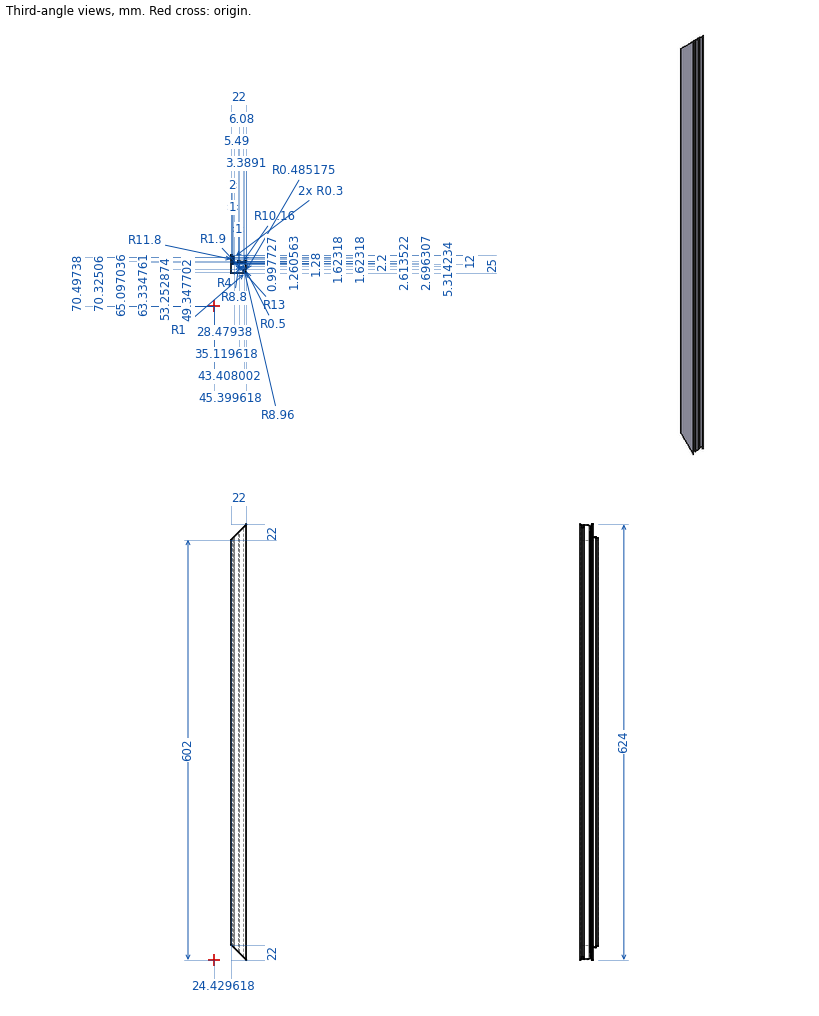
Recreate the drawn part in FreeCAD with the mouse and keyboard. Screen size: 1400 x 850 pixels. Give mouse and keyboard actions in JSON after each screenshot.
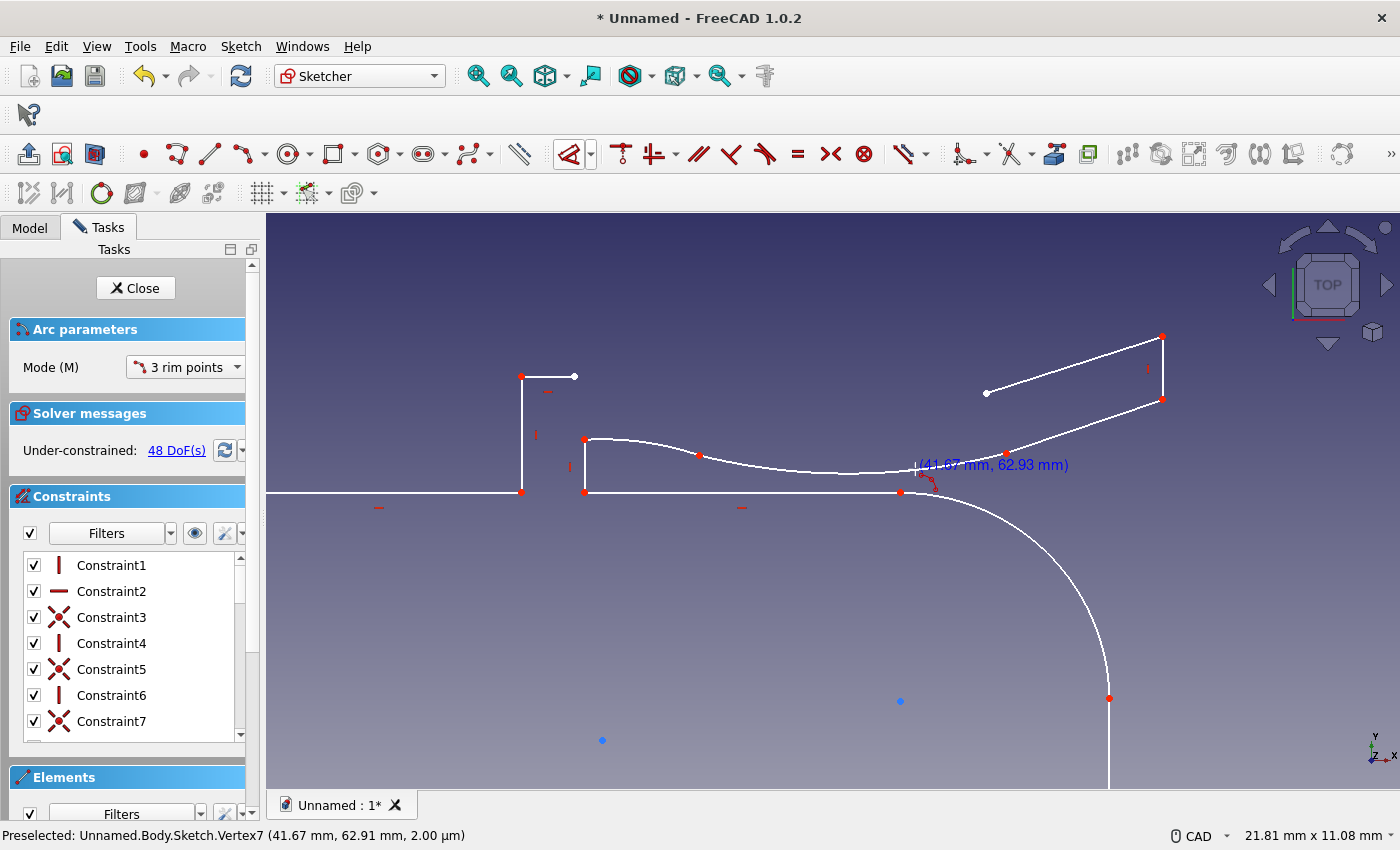
{"action": "left_click", "coordinate": [987, 393]}
{"action": "left_click", "coordinate": [717, 394]}
{"action": "left_click", "coordinate": [852, 412]}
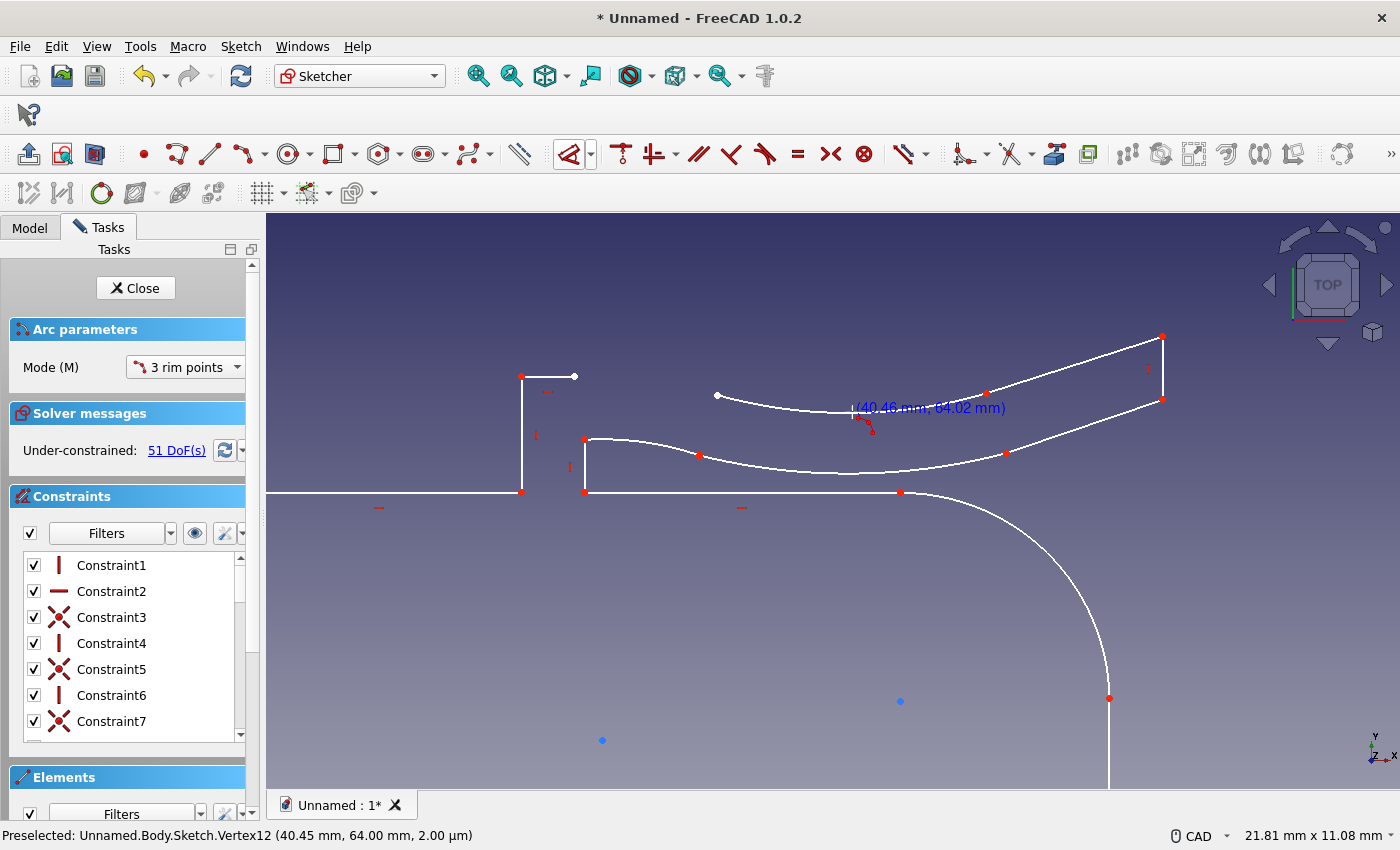
{"action": "left_click", "coordinate": [717, 395]}
{"action": "left_click", "coordinate": [575, 377]}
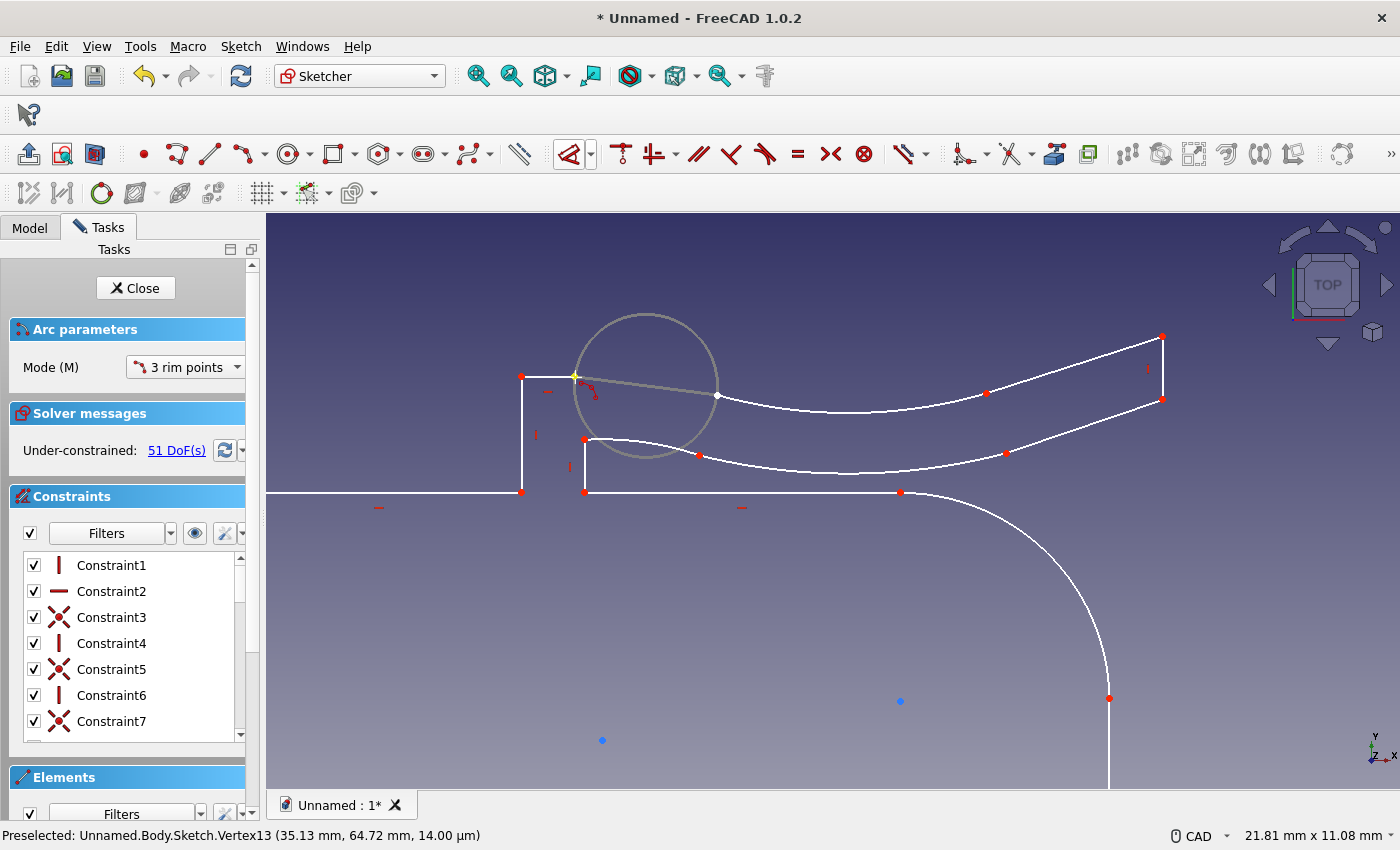
{"action": "scroll", "coordinate": [646, 379], "scroll_direction": "up", "scroll_amount": 6}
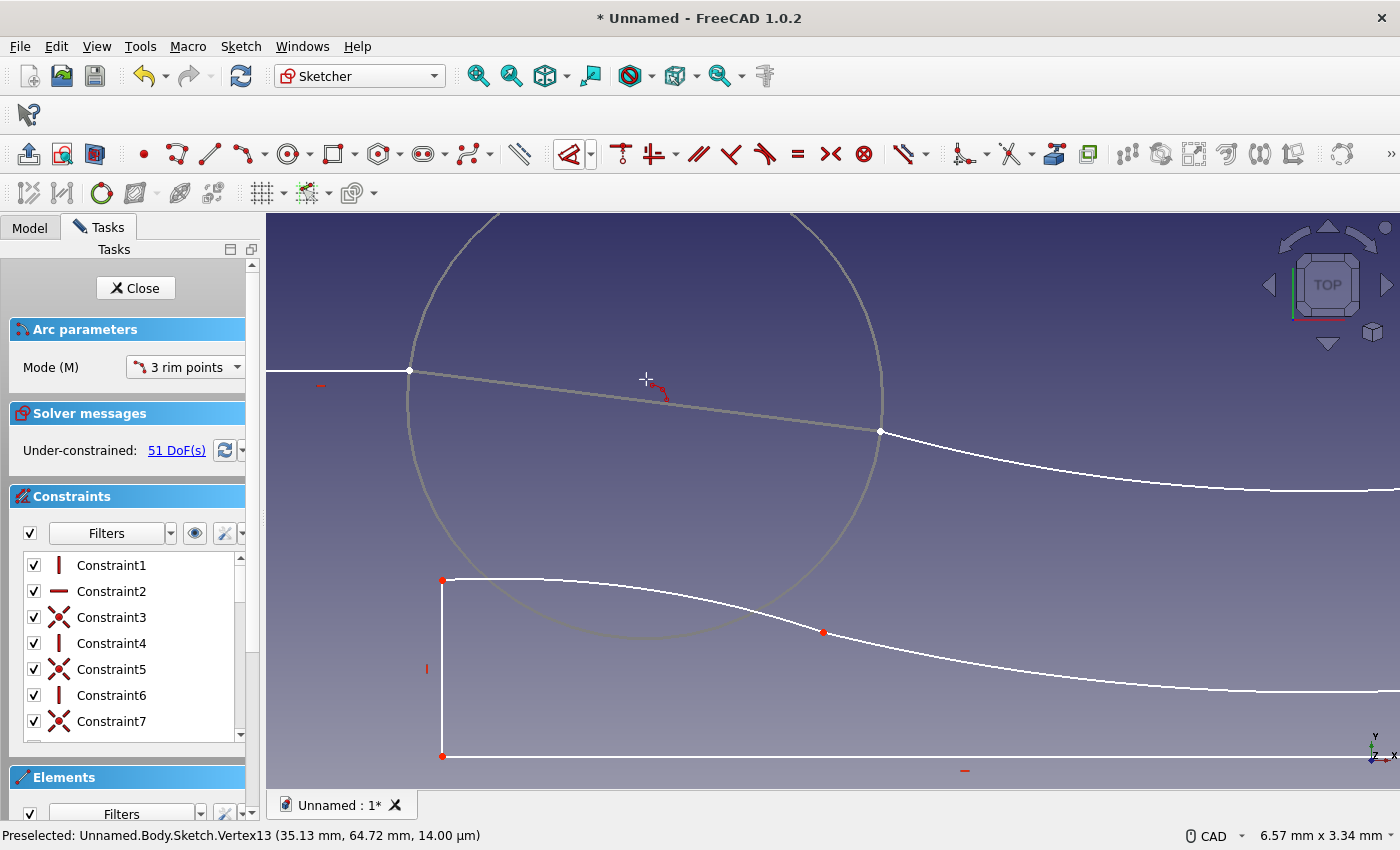
{"action": "left_click", "coordinate": [646, 379]}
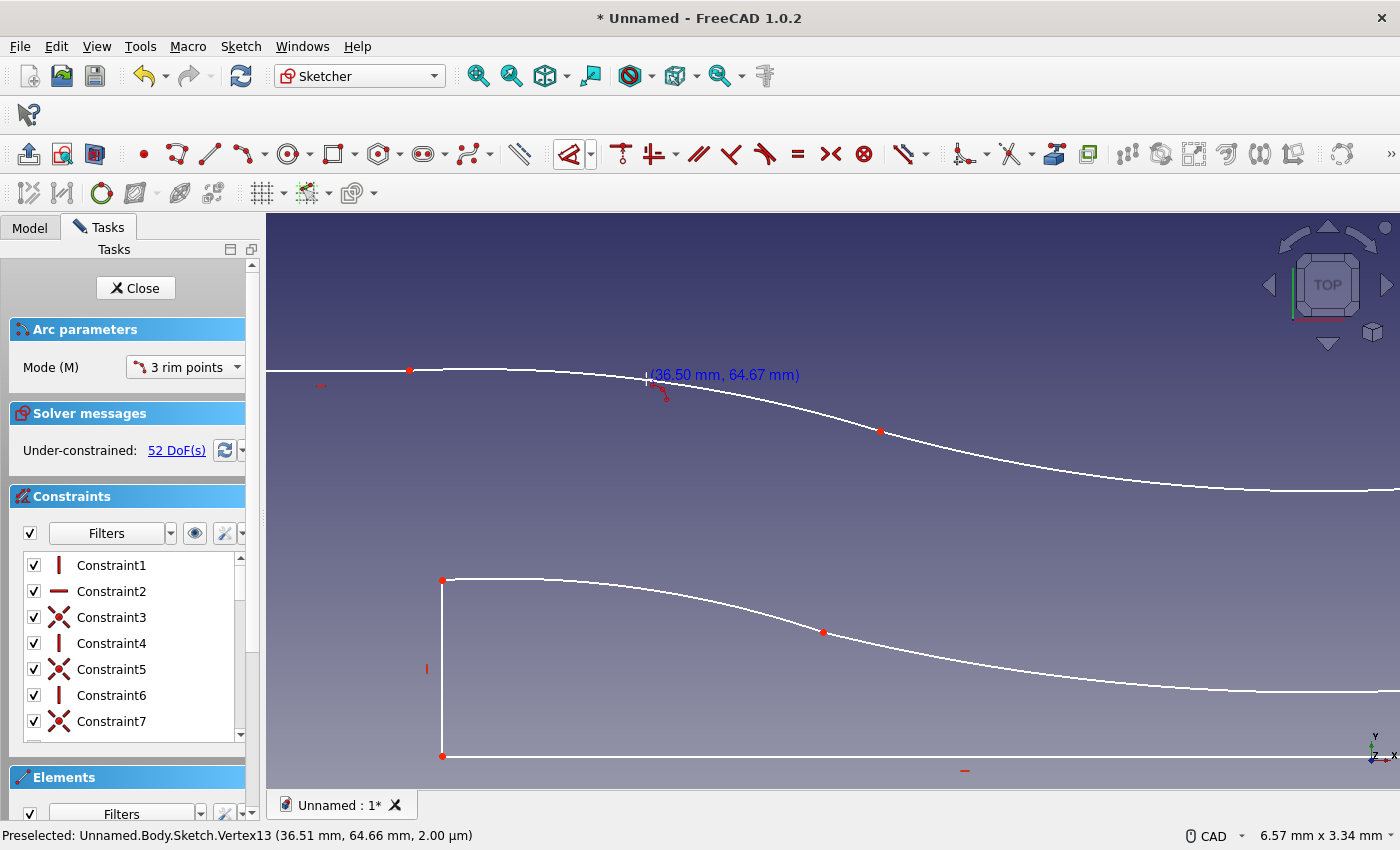
{"action": "scroll", "coordinate": [795, 445], "scroll_direction": "down", "scroll_amount": 12}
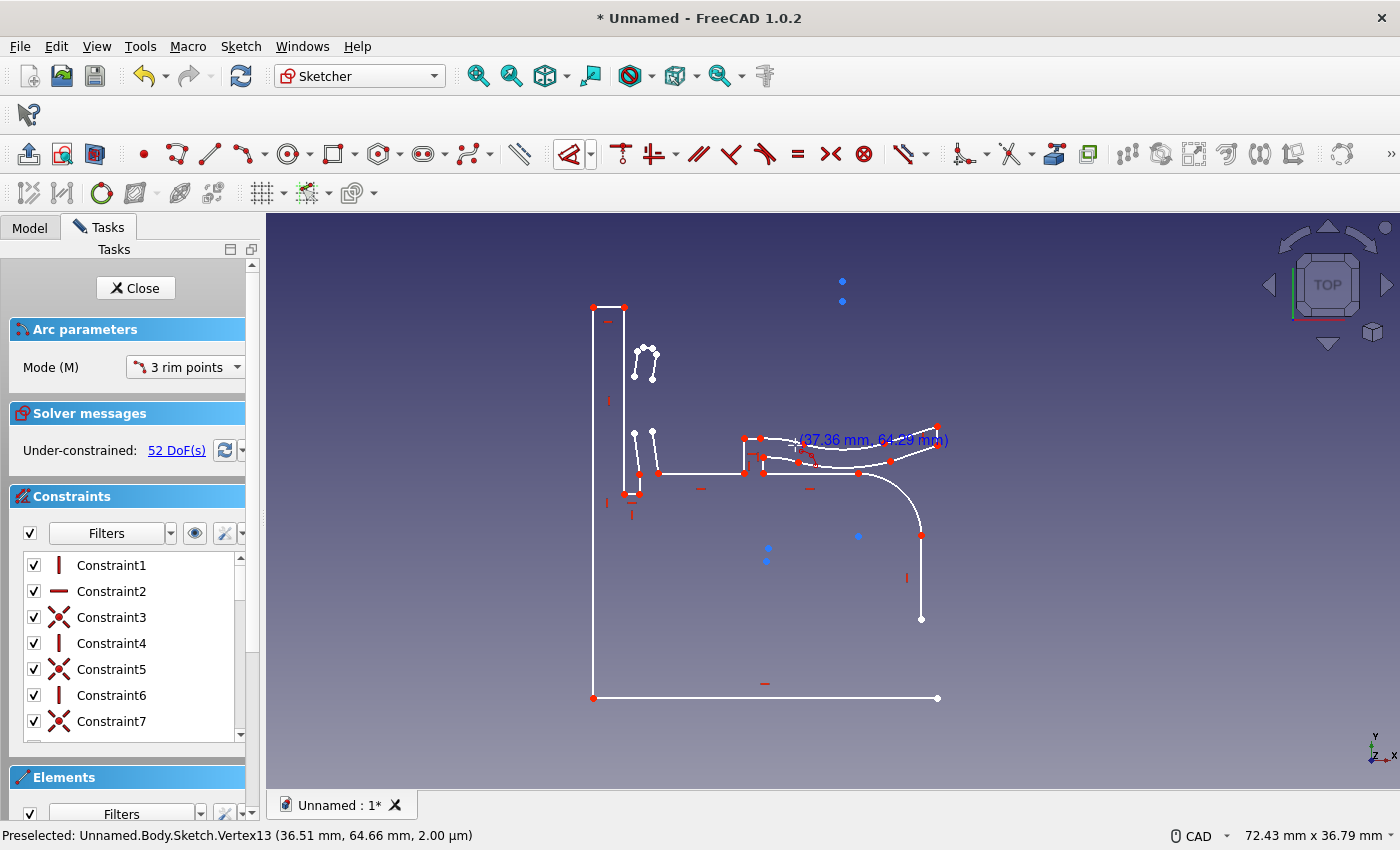
{"action": "left_click", "coordinate": [652, 432]}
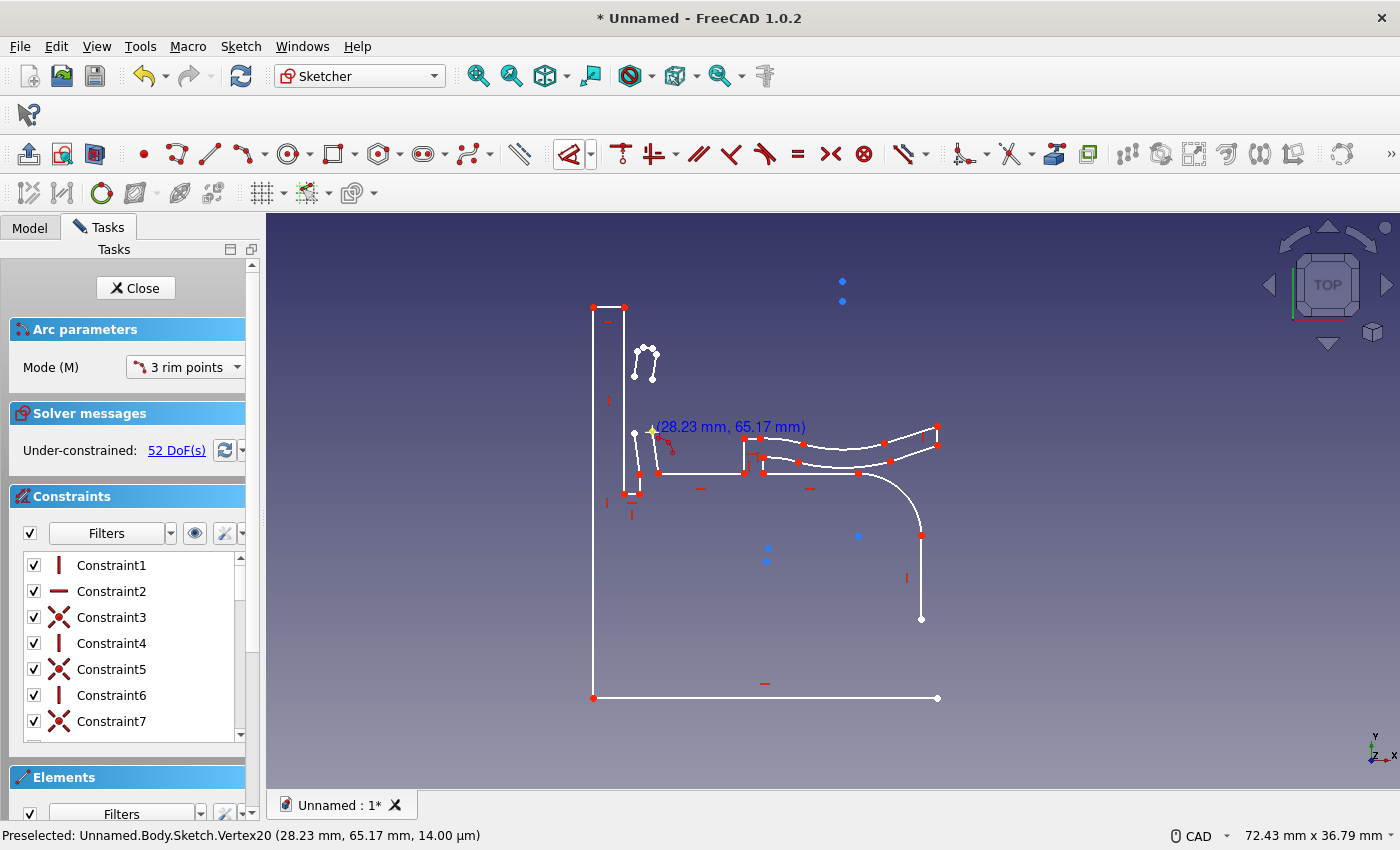
{"action": "scroll", "coordinate": [653, 379], "scroll_direction": "up", "scroll_amount": 2}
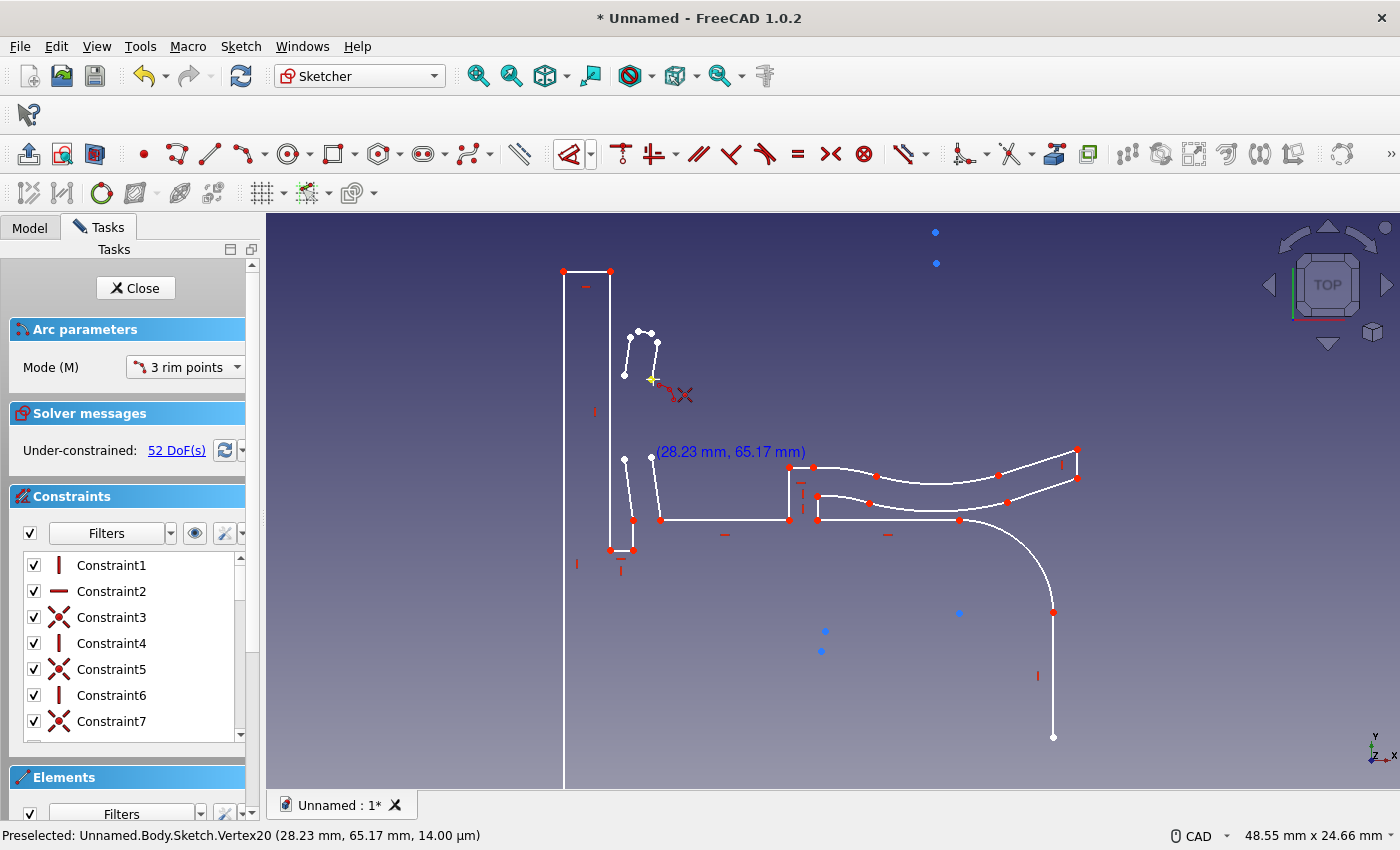
{"action": "left_click", "coordinate": [652, 380]}